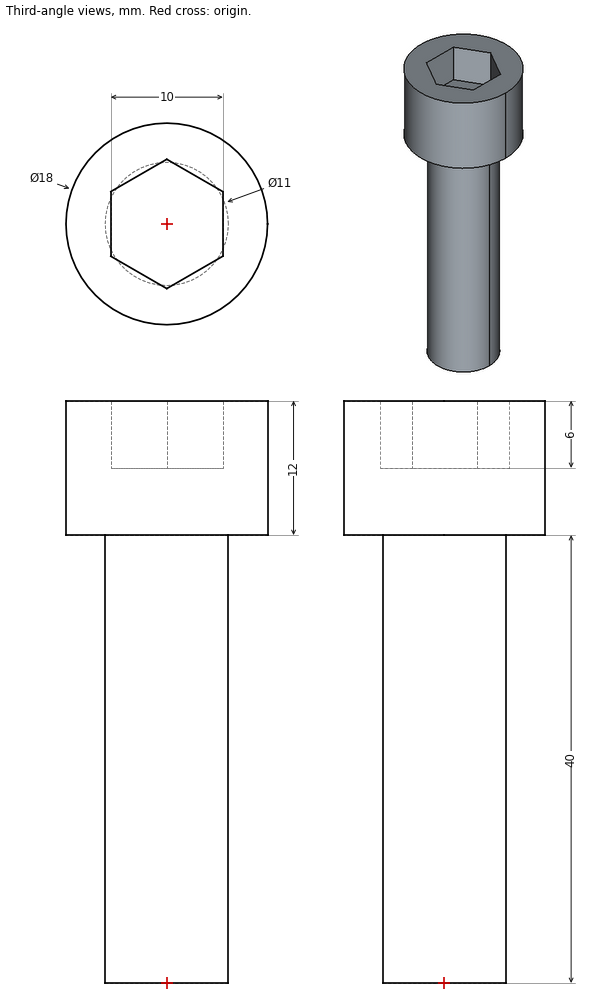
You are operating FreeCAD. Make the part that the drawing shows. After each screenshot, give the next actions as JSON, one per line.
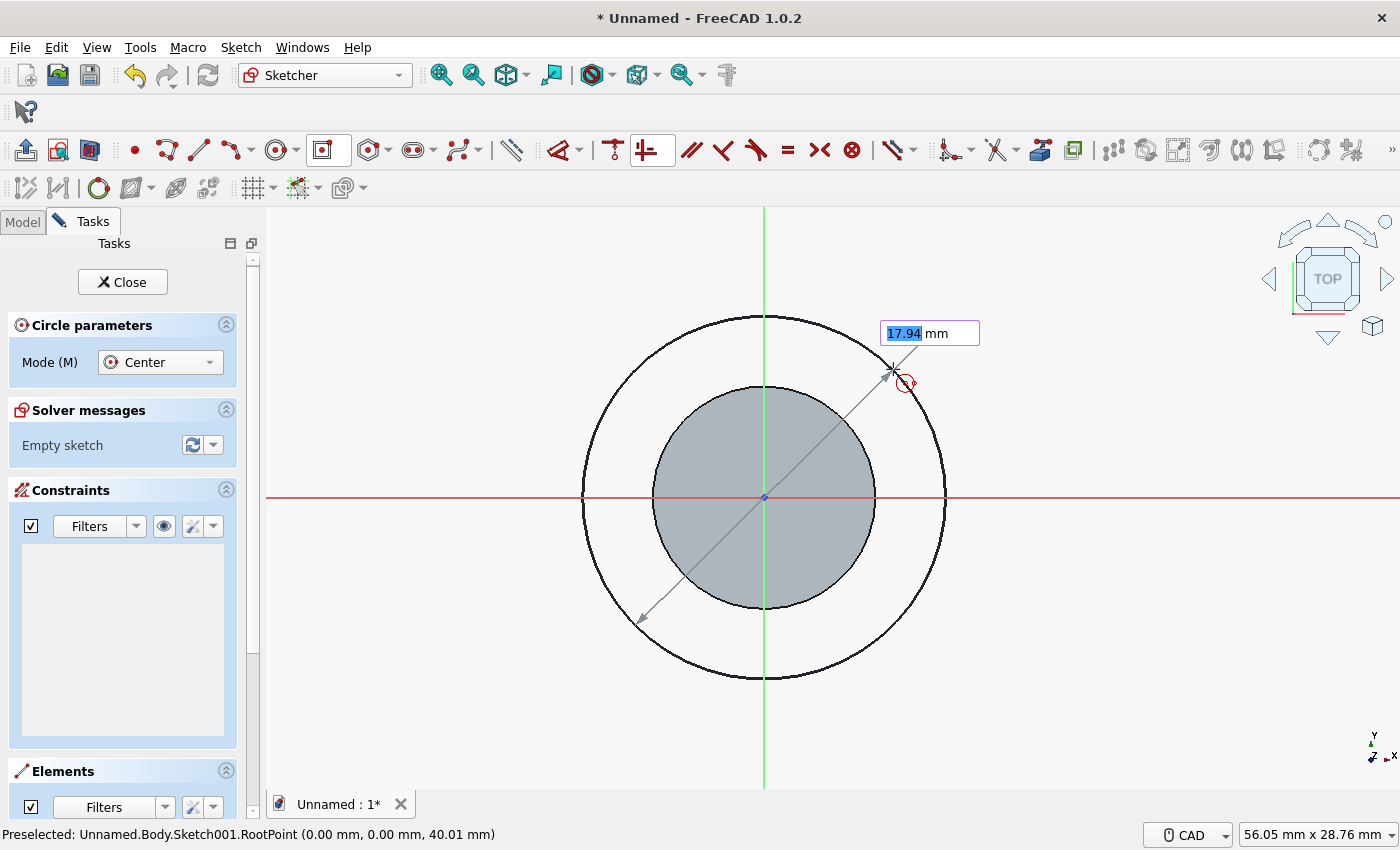
{"action": "type", "text": "18"}
{"action": "key", "text": "Return"}
{"action": "key", "text": "Escape"}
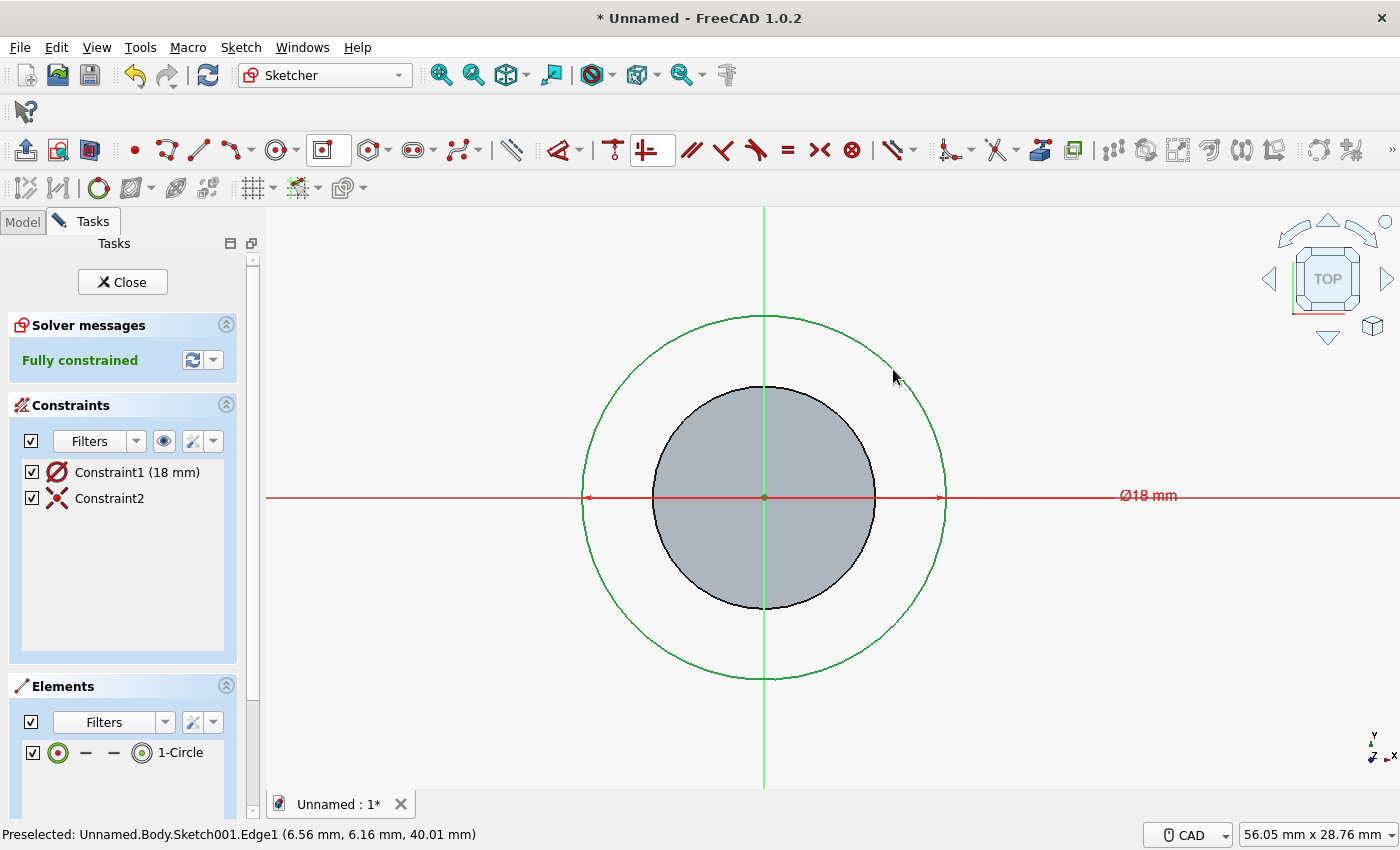
{"action": "left_click", "coordinate": [123, 282]}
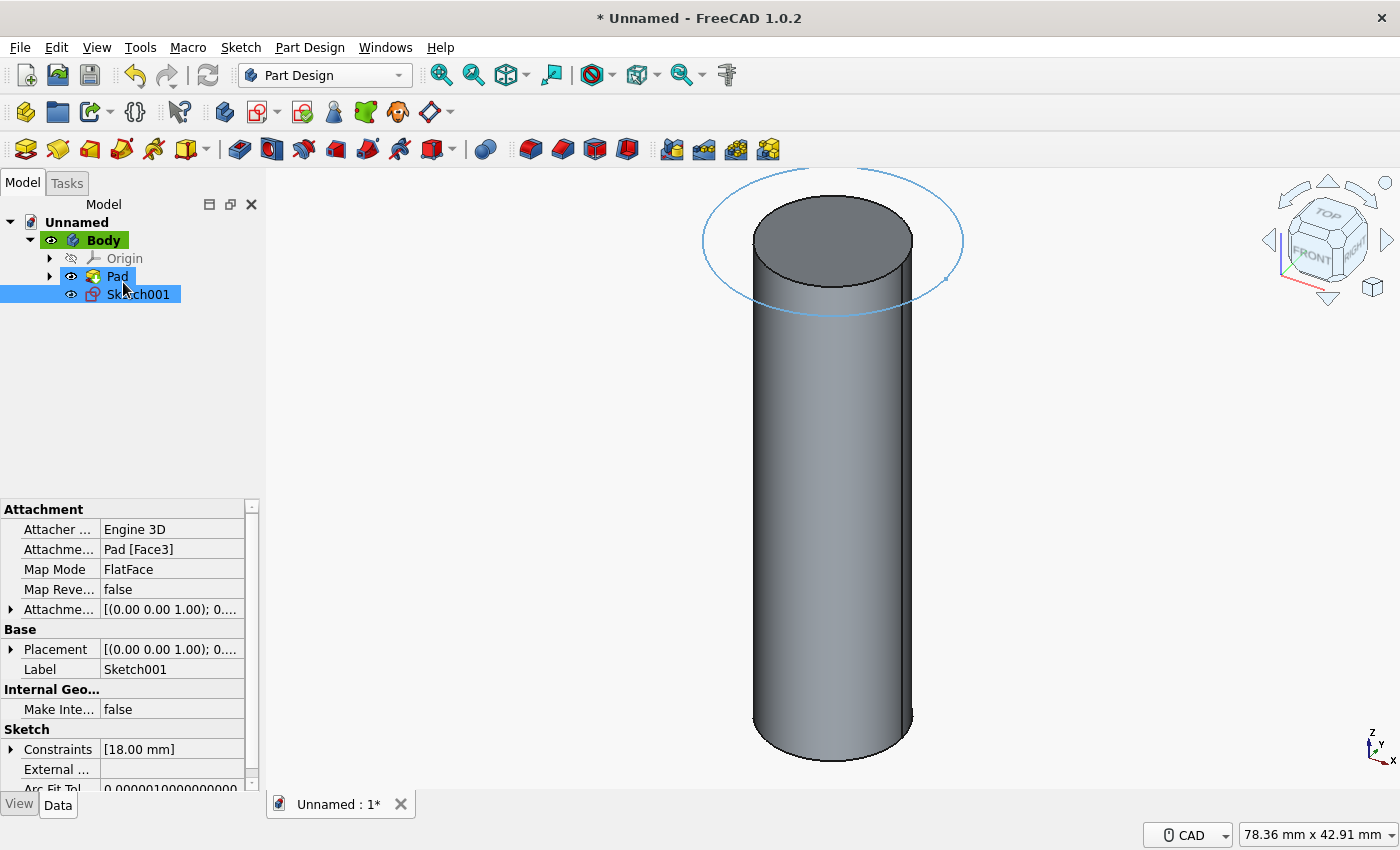
{"action": "left_click", "coordinate": [26, 150]}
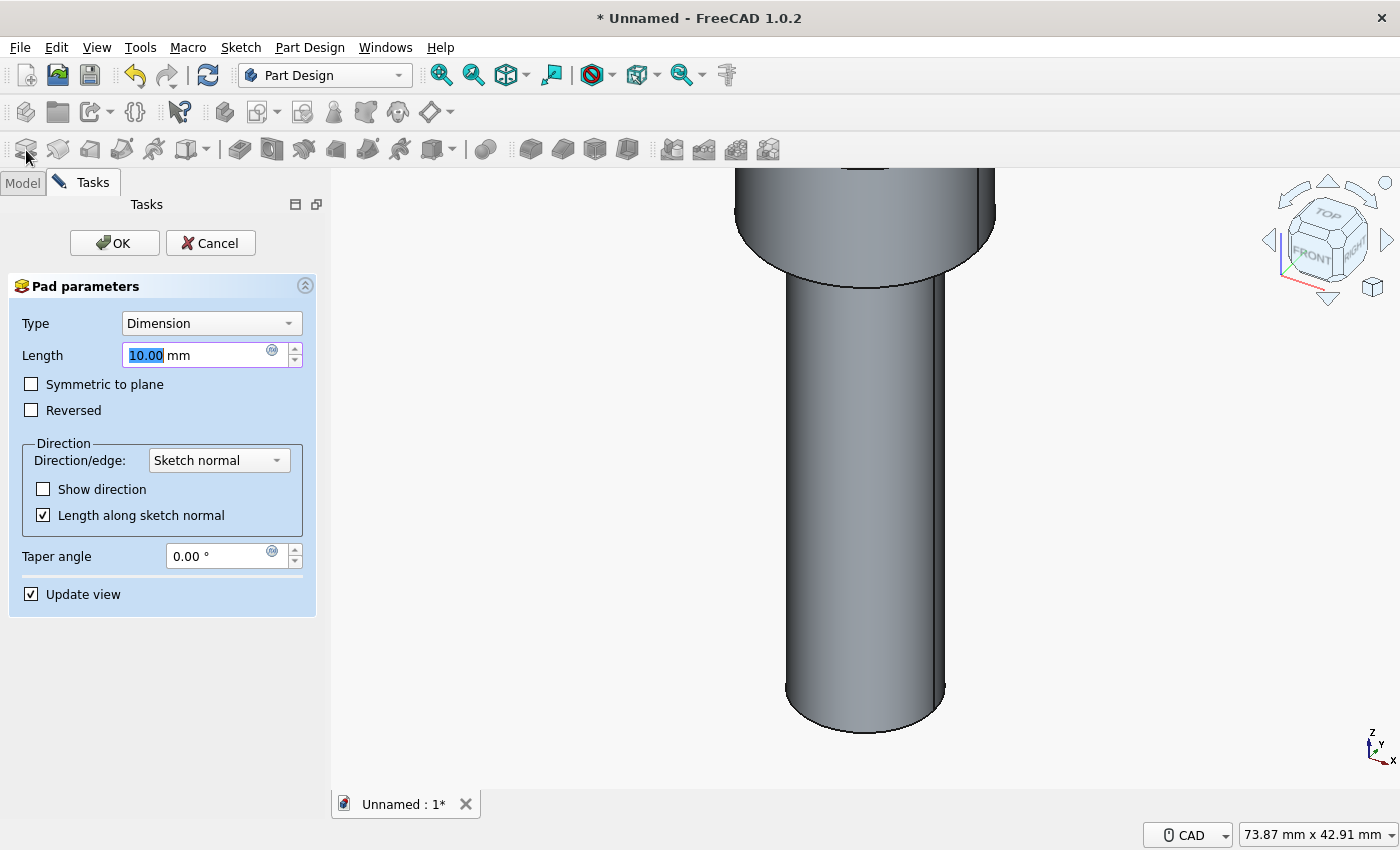
{"action": "type", "text": "12"}
{"action": "key", "text": "Tab"}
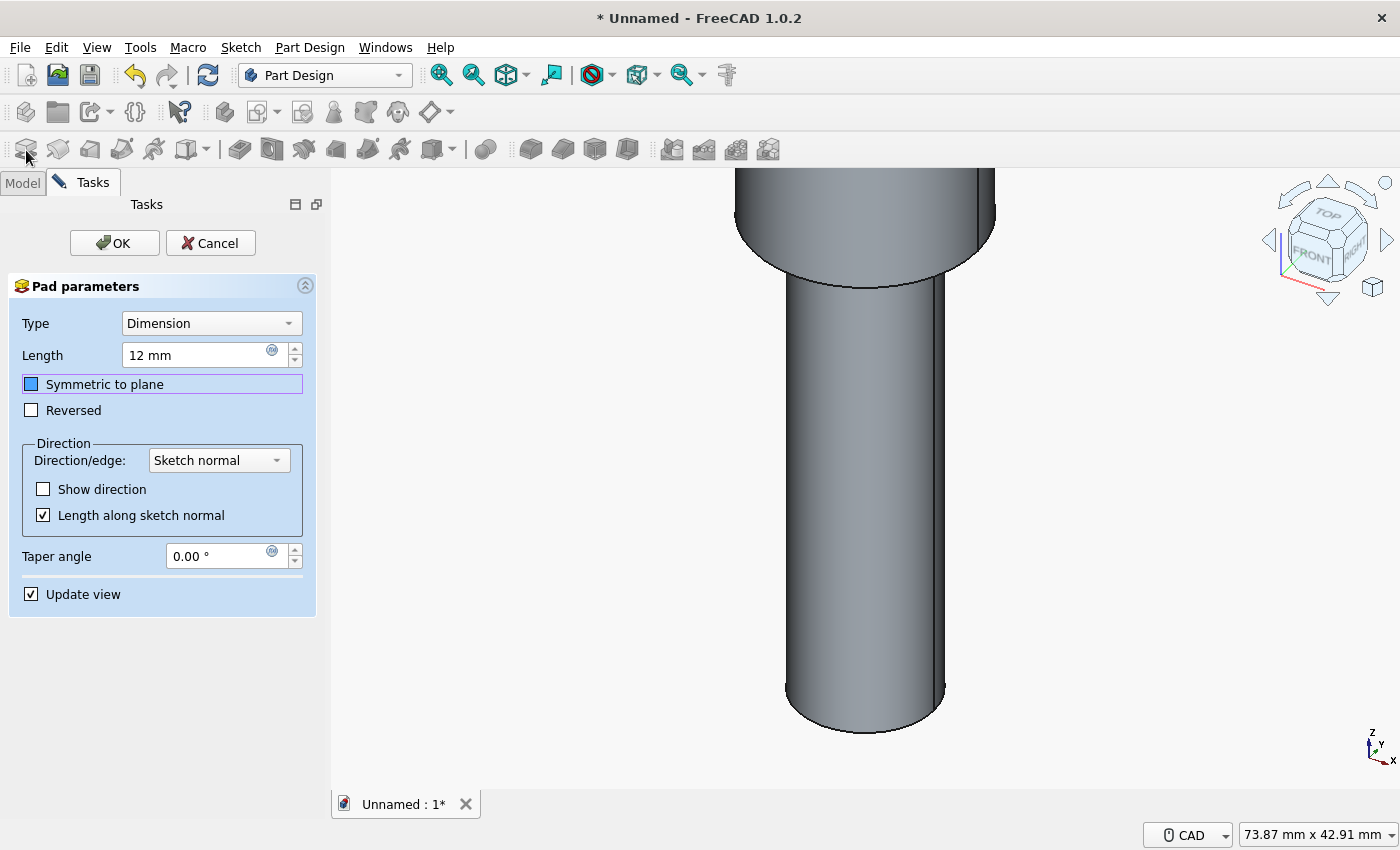
{"action": "left_click", "coordinate": [115, 243]}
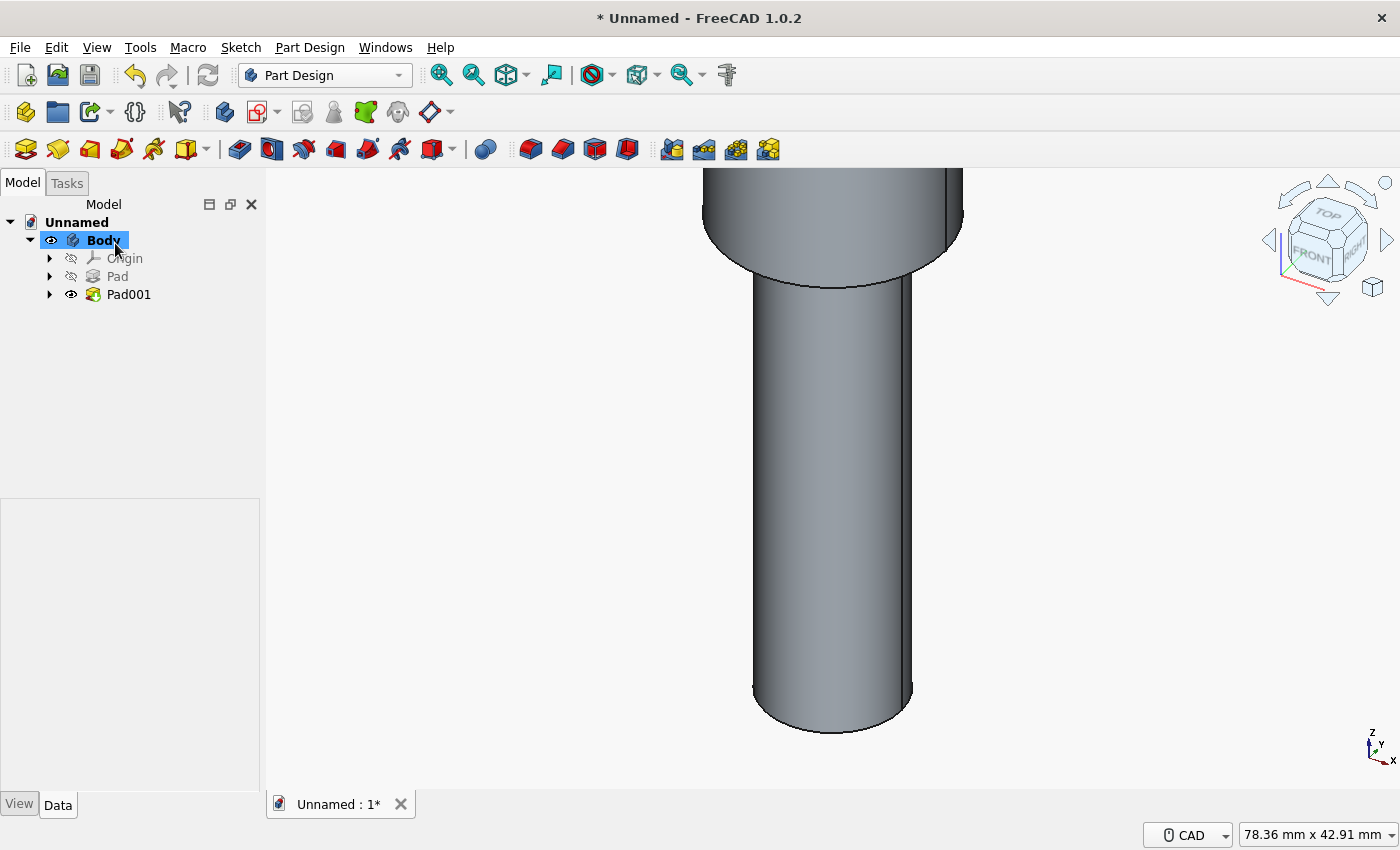
{"action": "left_click", "coordinate": [442, 76]}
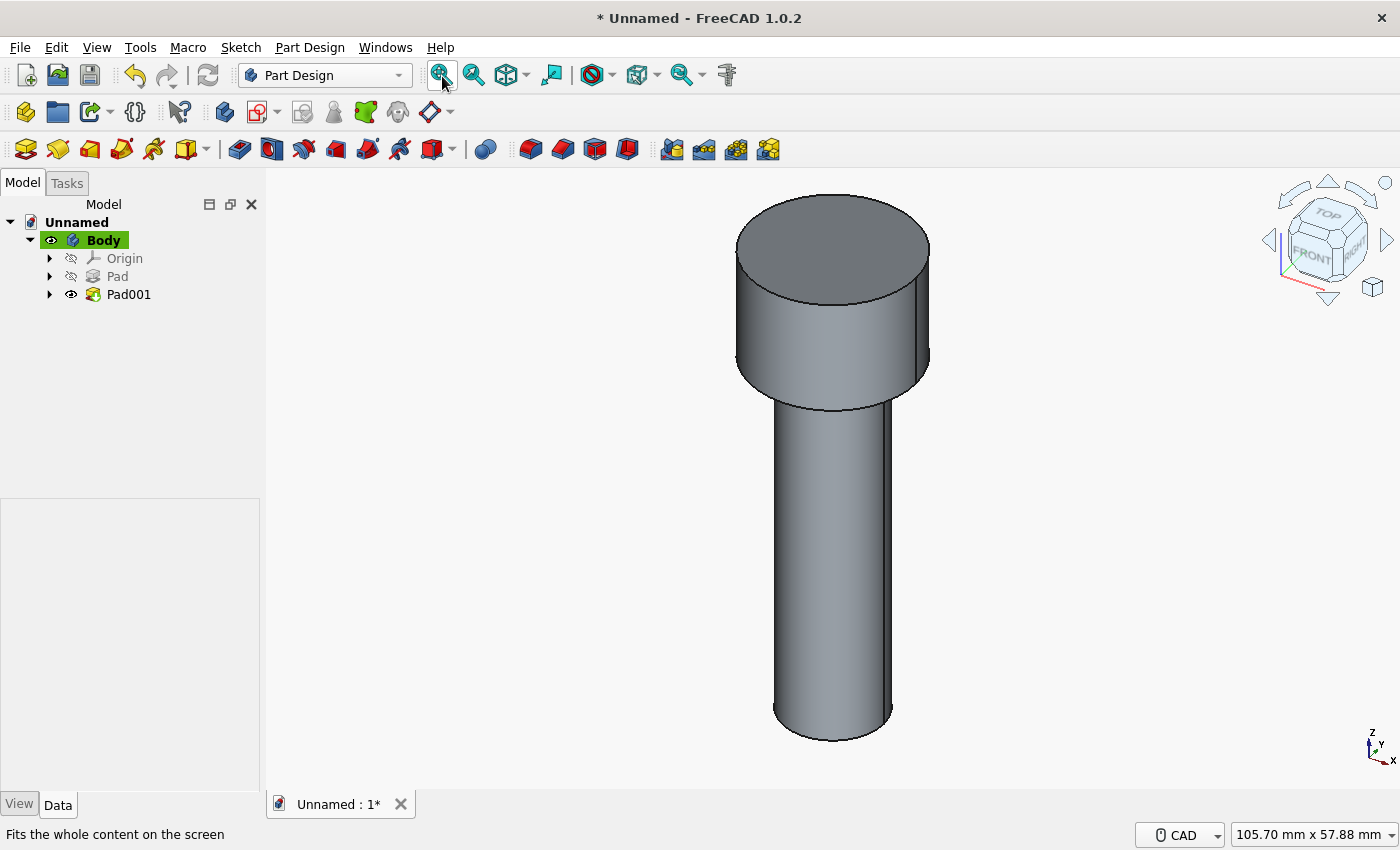
{"action": "left_click", "coordinate": [833, 249]}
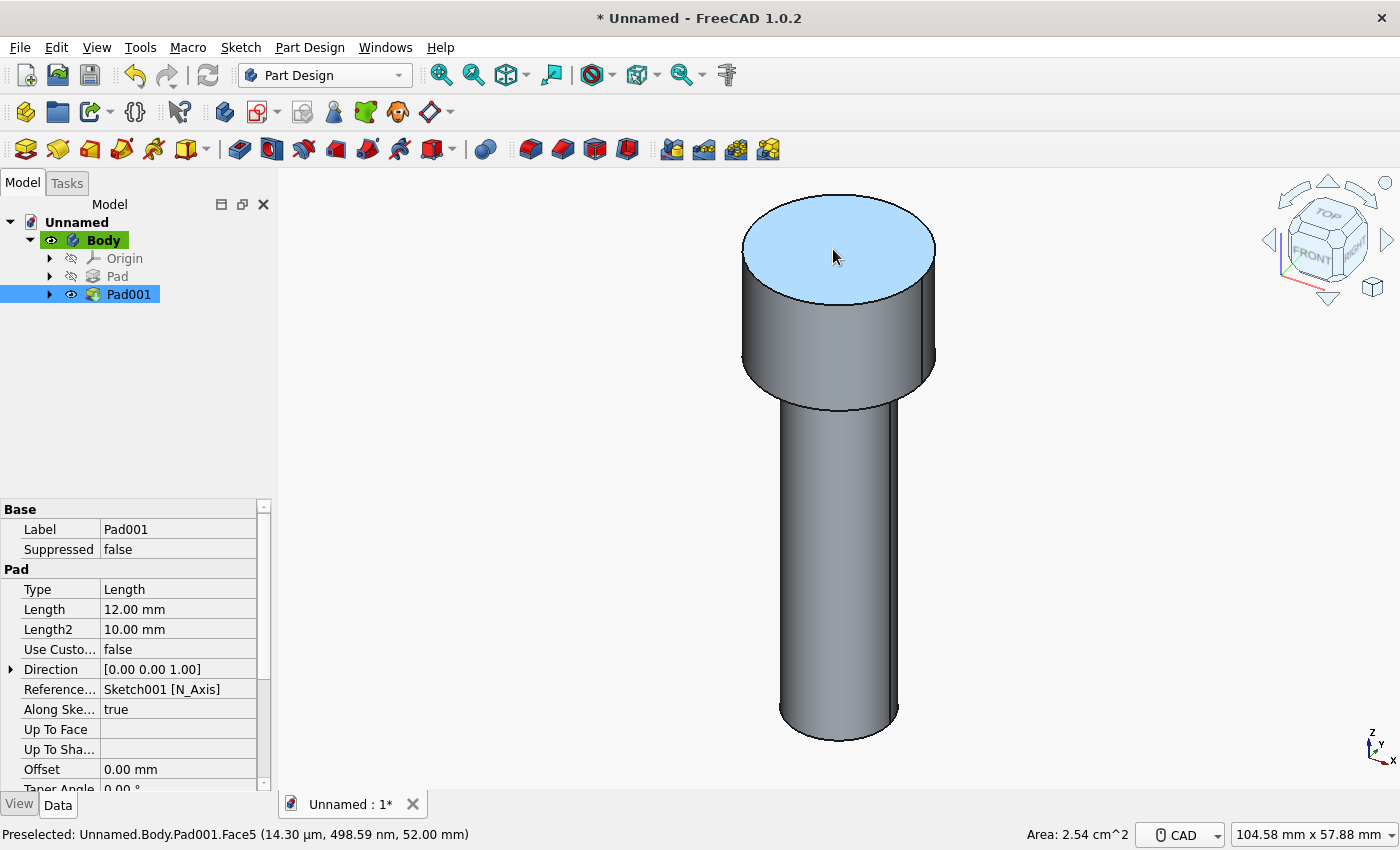
{"action": "left_click", "coordinate": [258, 112]}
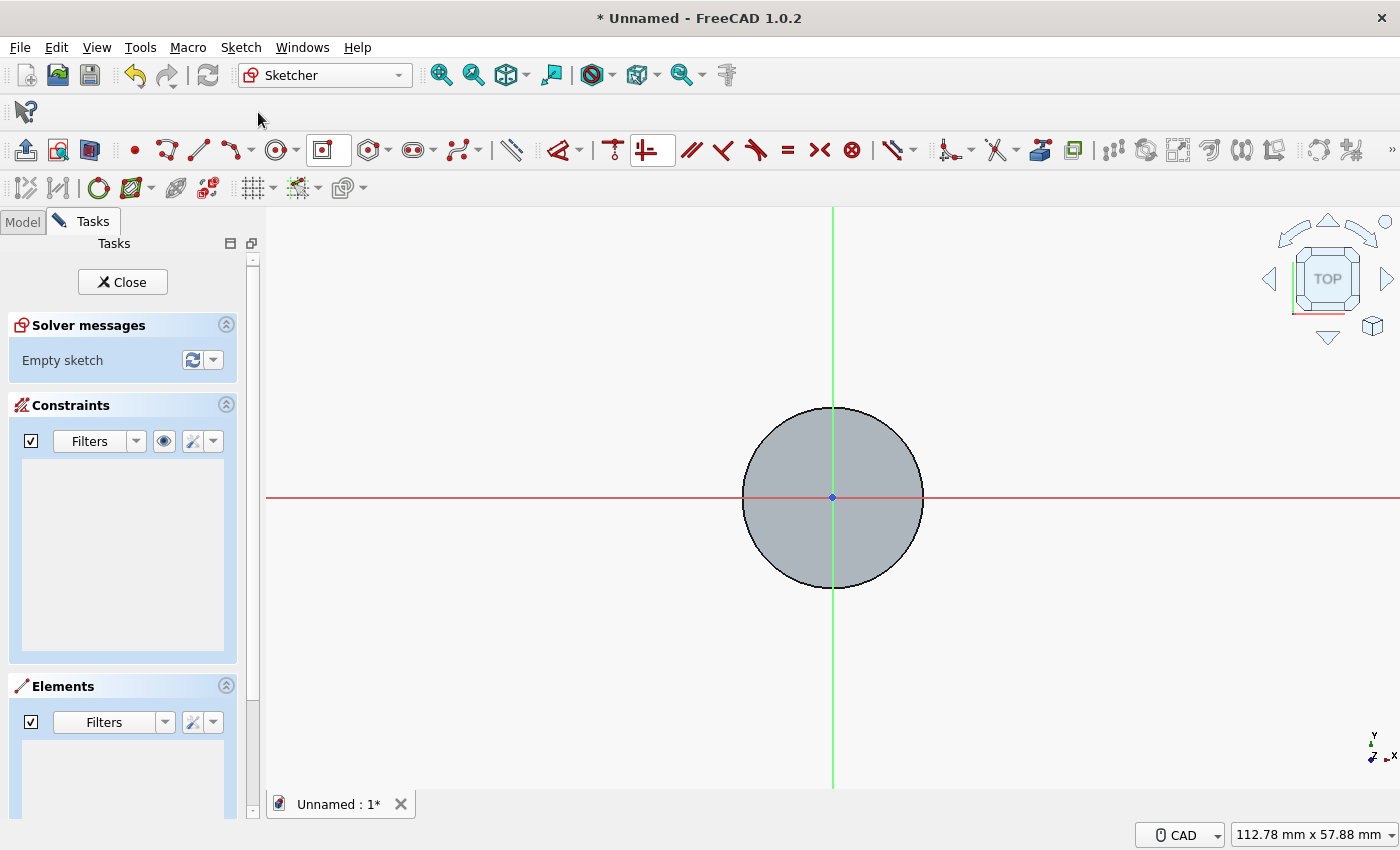
{"action": "scroll", "coordinate": [862, 498], "scroll_direction": "up", "scroll_amount": 6}